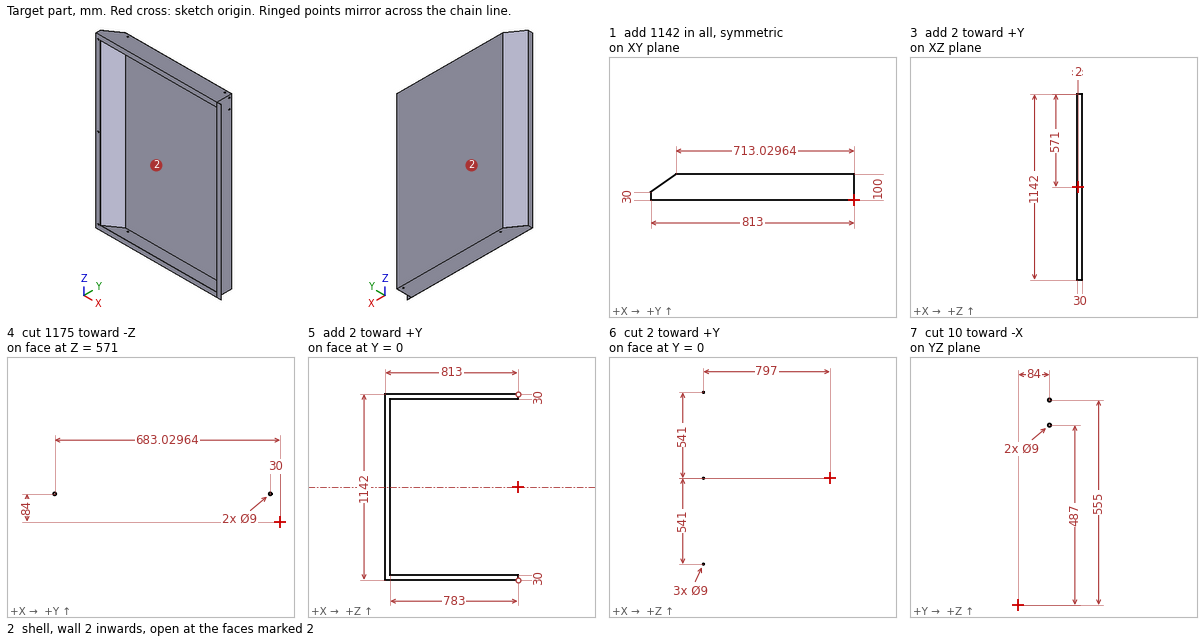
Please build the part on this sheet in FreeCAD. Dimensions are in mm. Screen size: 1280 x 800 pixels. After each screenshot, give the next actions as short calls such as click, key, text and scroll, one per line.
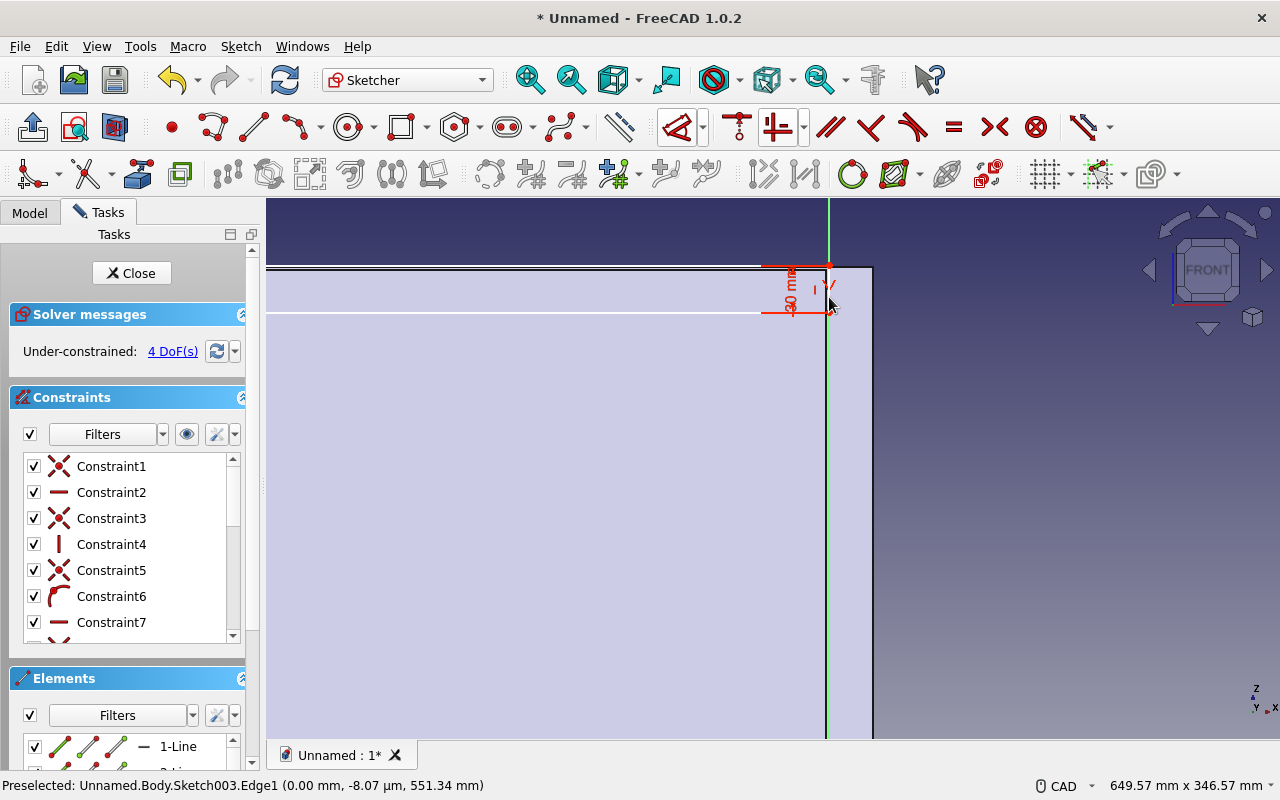
scroll(834, 294, down, 8)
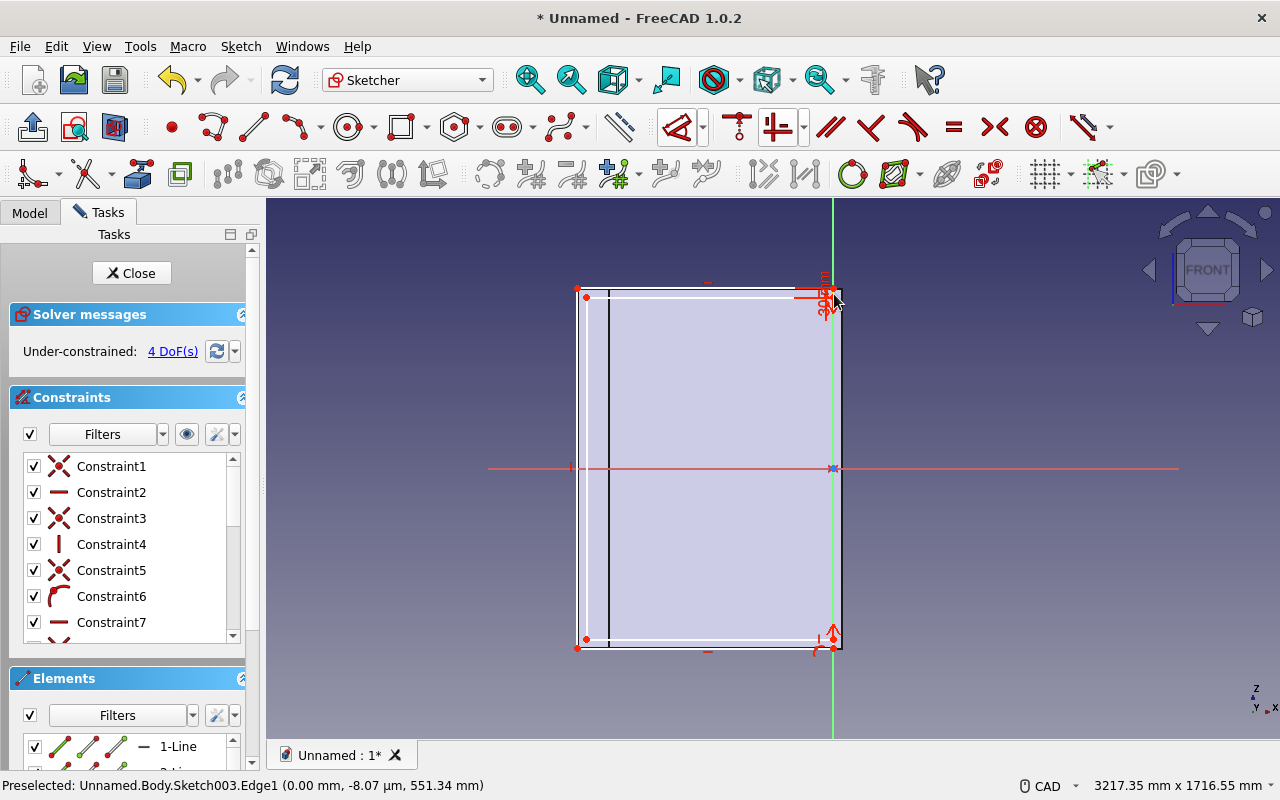
scroll(833, 646, up, 8)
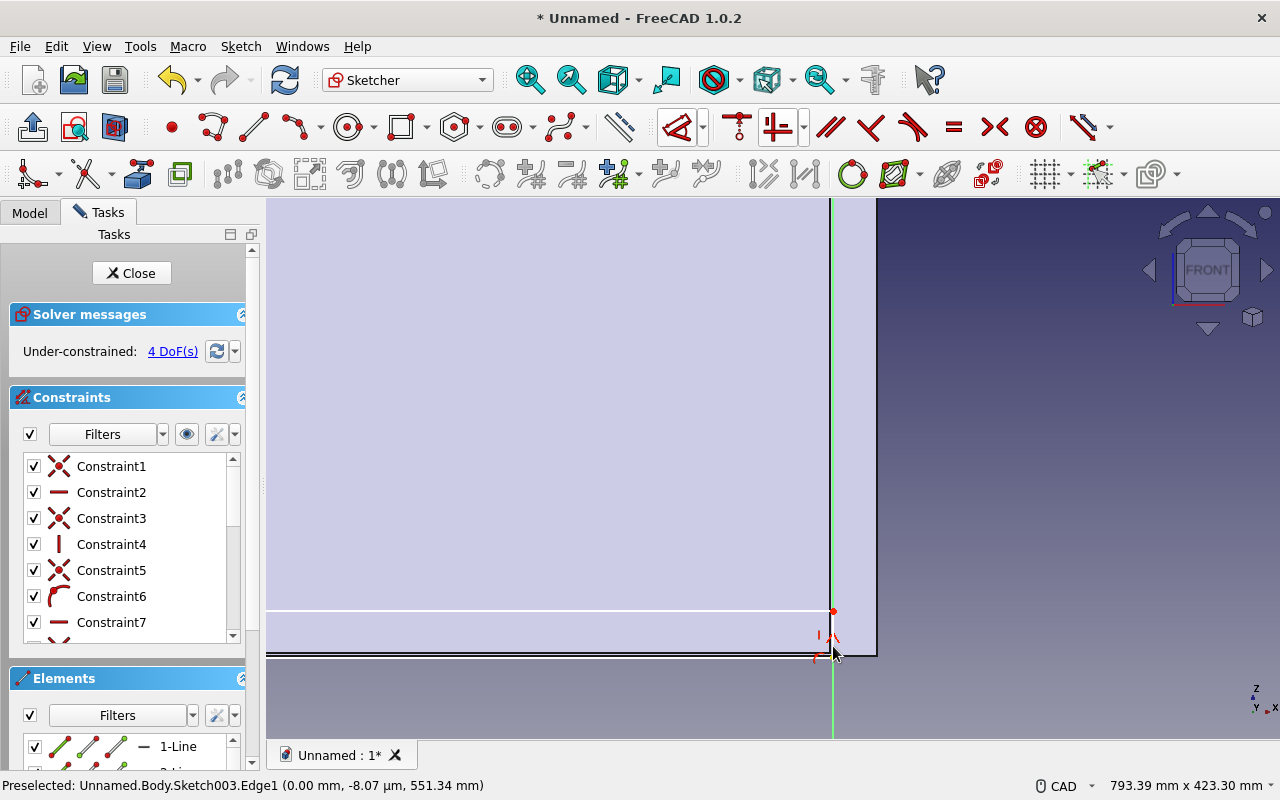
click(833, 644)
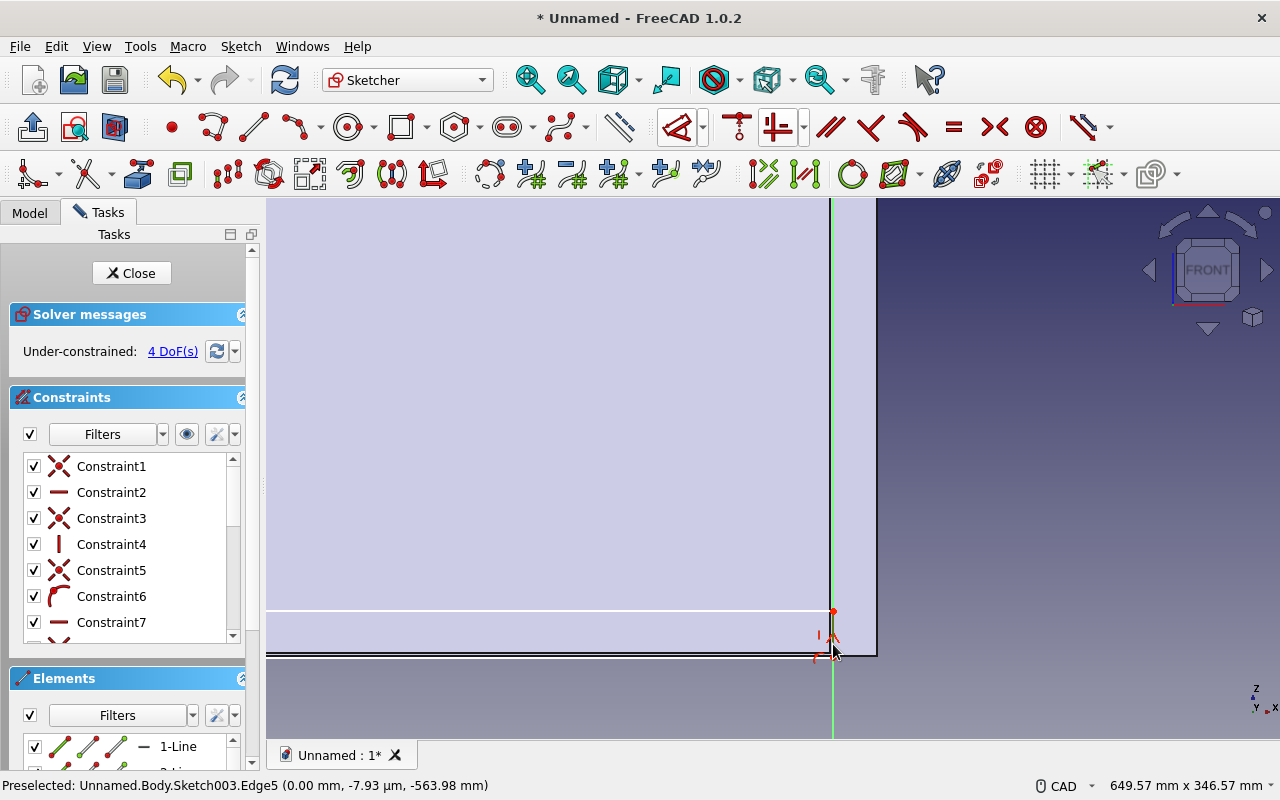
key(i)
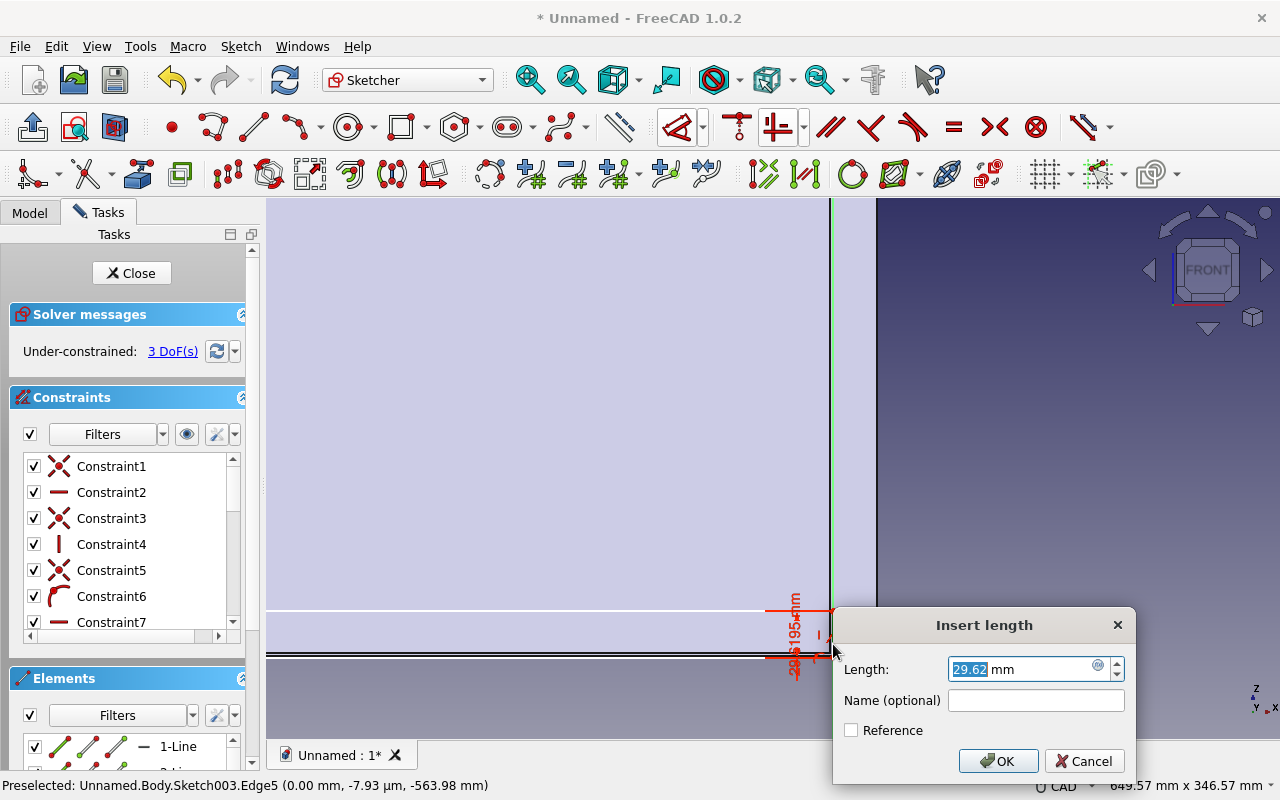
text(30)
key(Return)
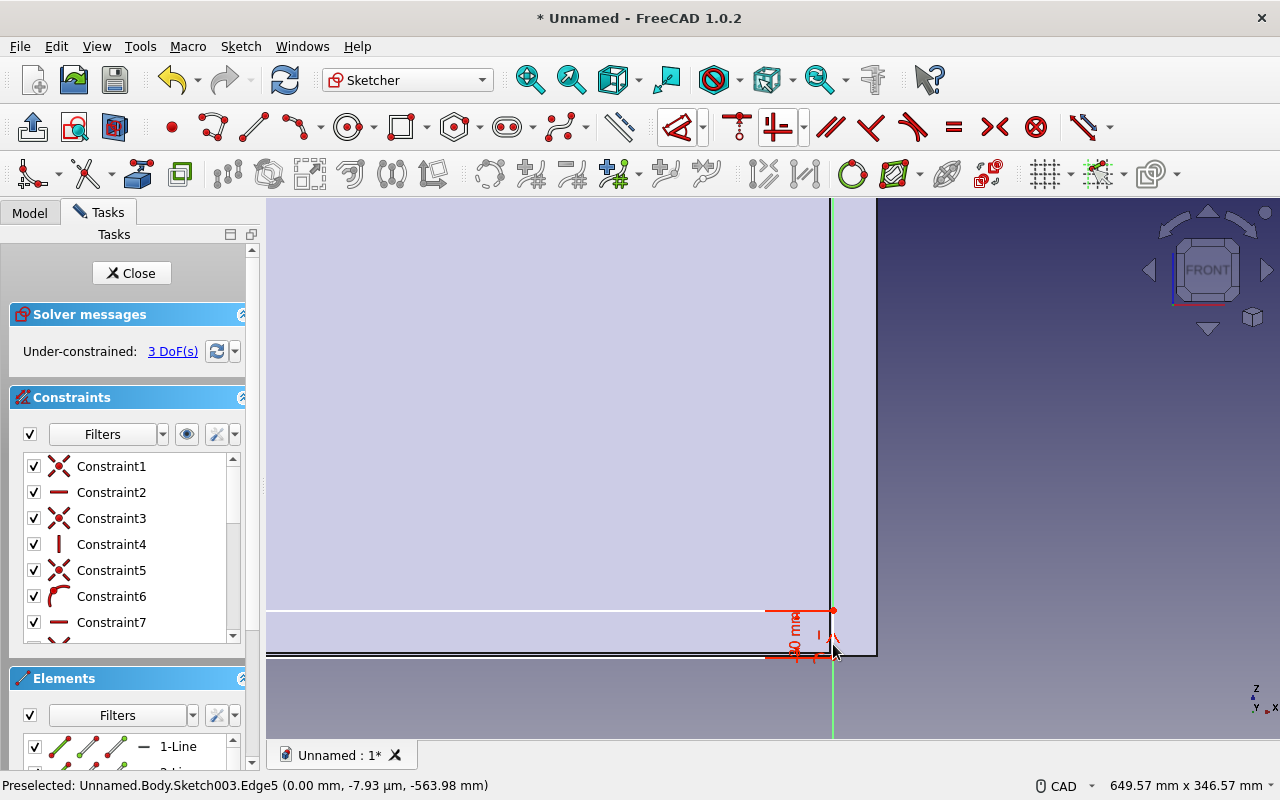
scroll(833, 647, down, 8)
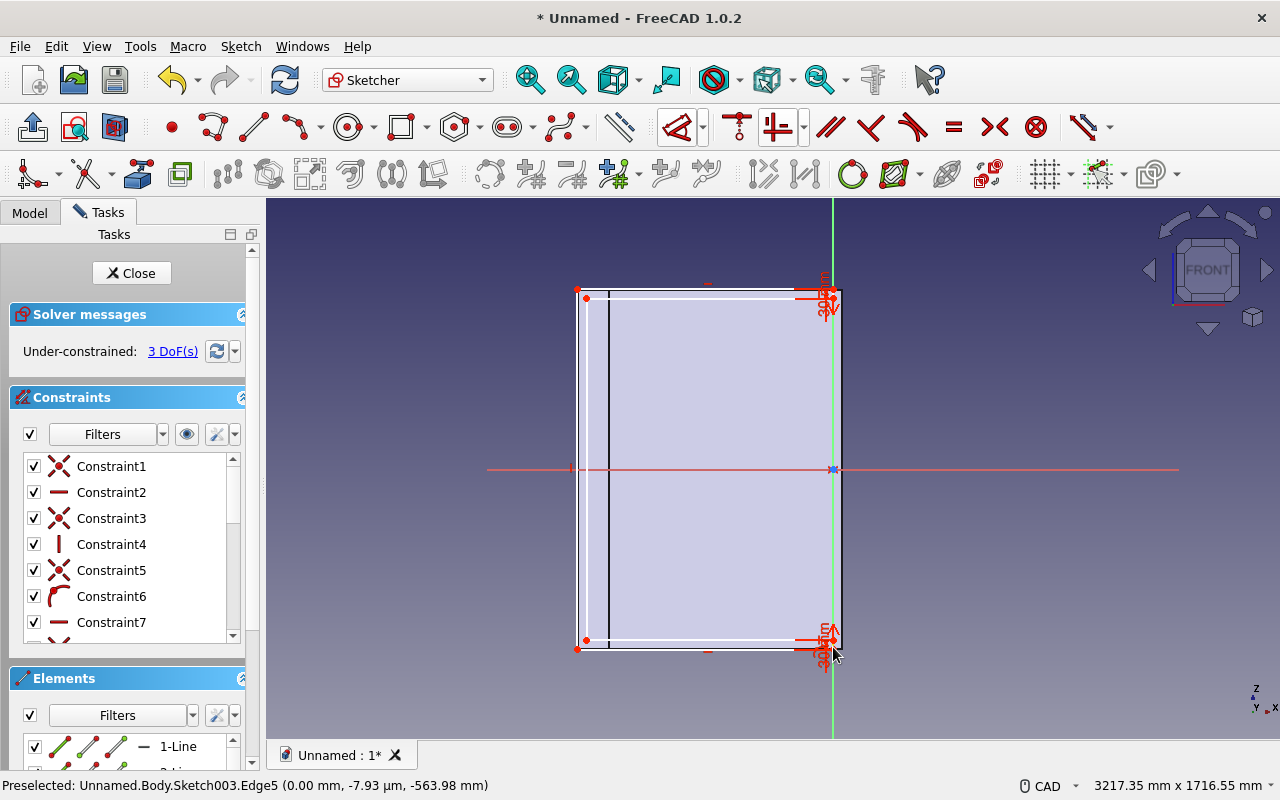
scroll(757, 289, up, 2)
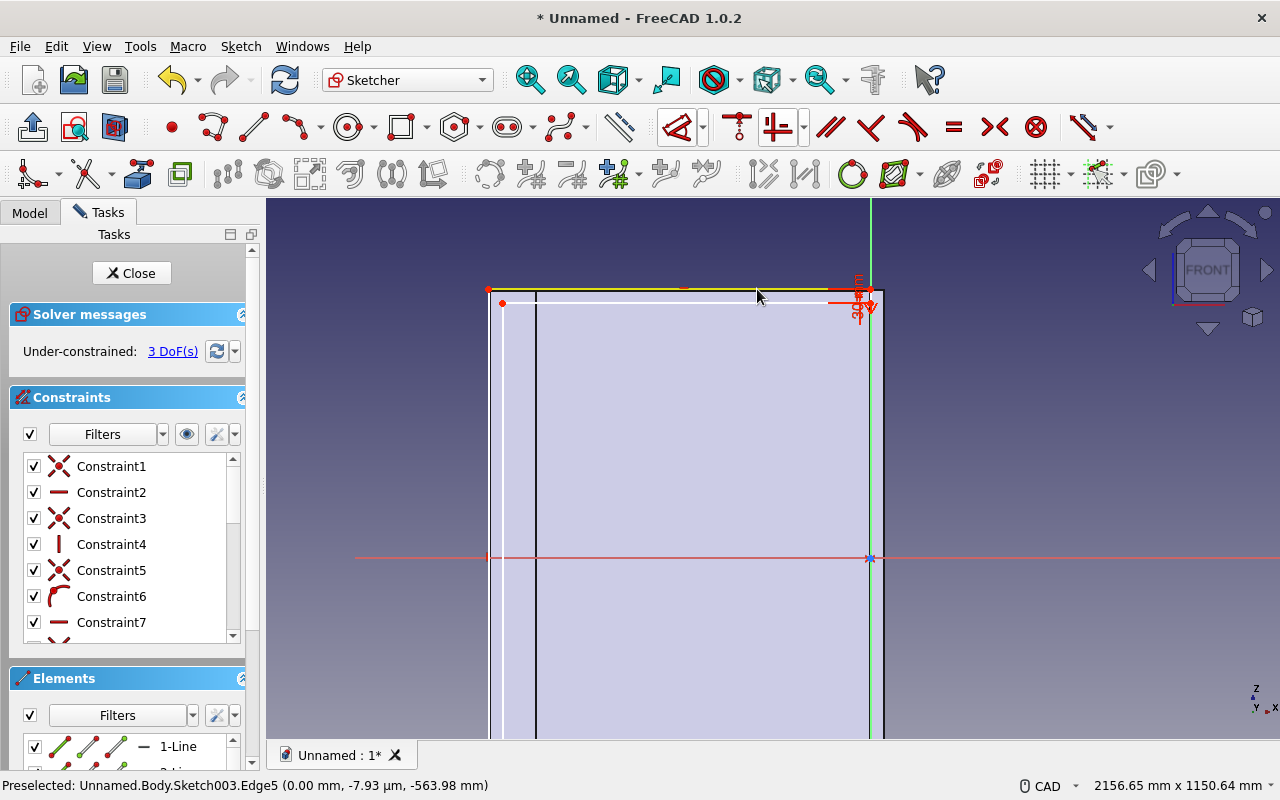
click(756, 289)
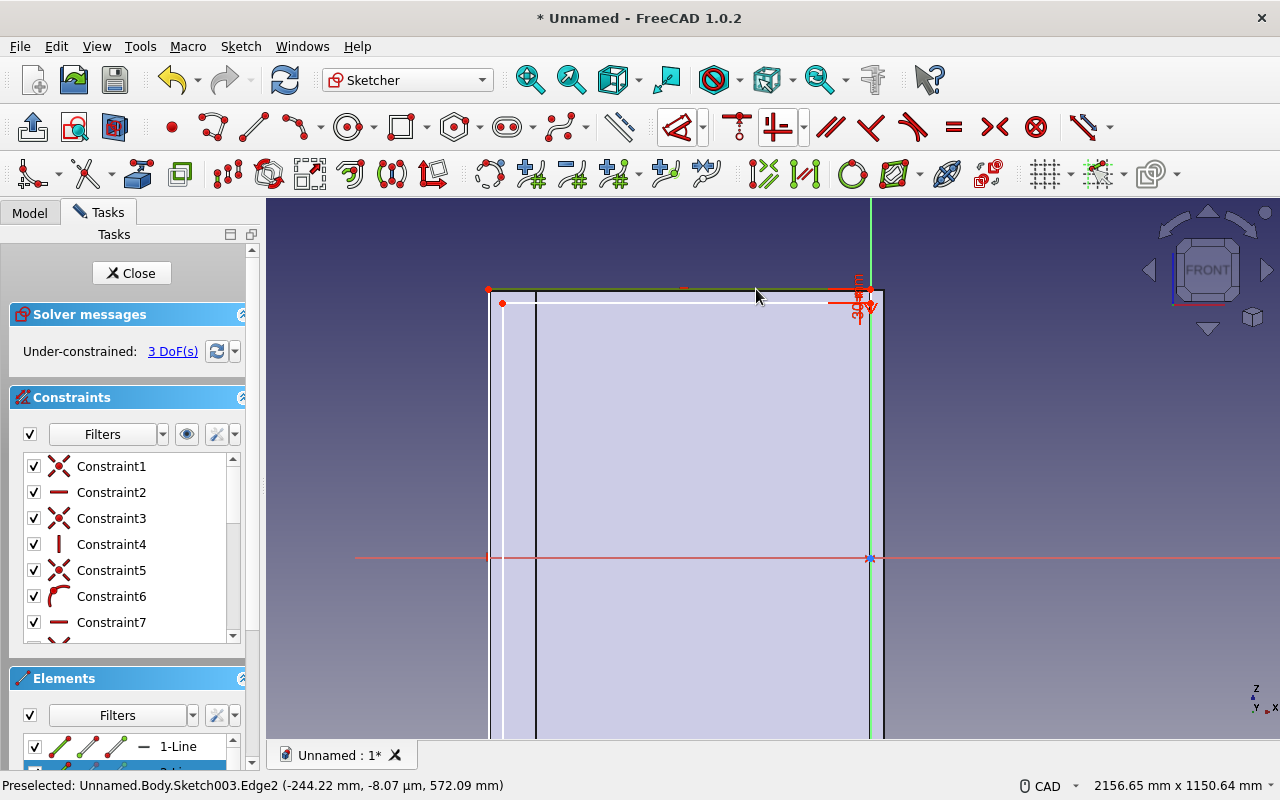
click(702, 128)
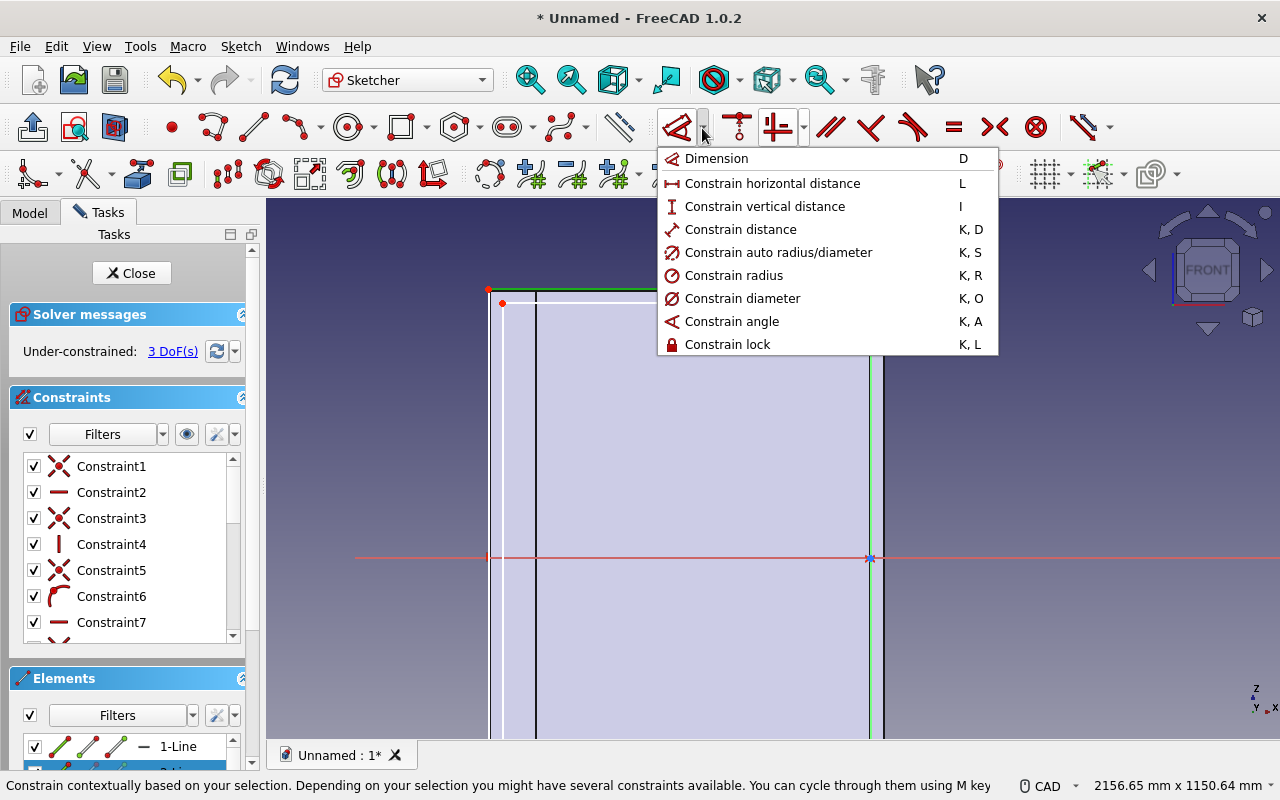
click(828, 184)